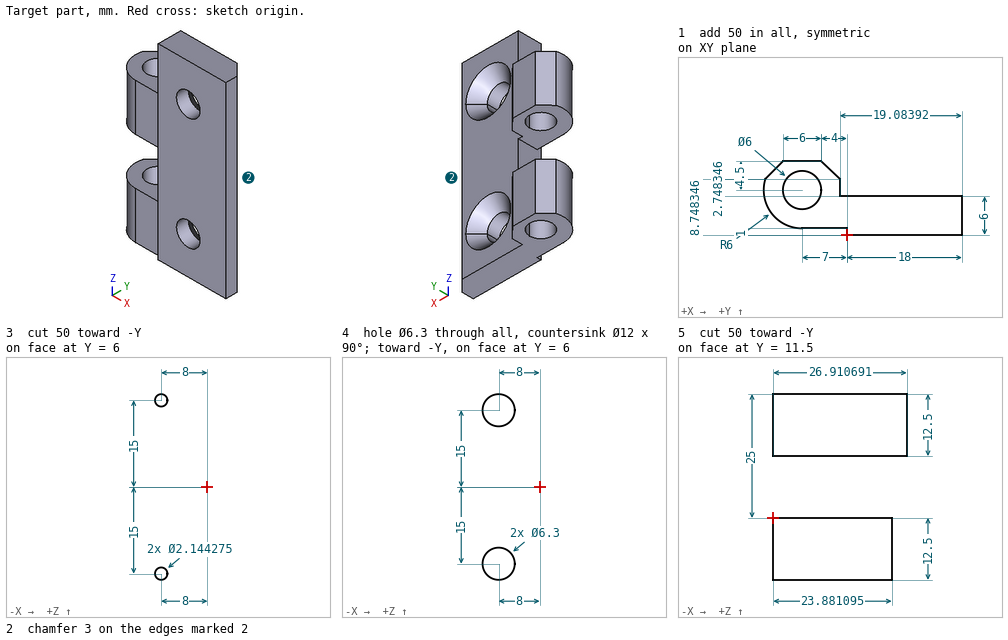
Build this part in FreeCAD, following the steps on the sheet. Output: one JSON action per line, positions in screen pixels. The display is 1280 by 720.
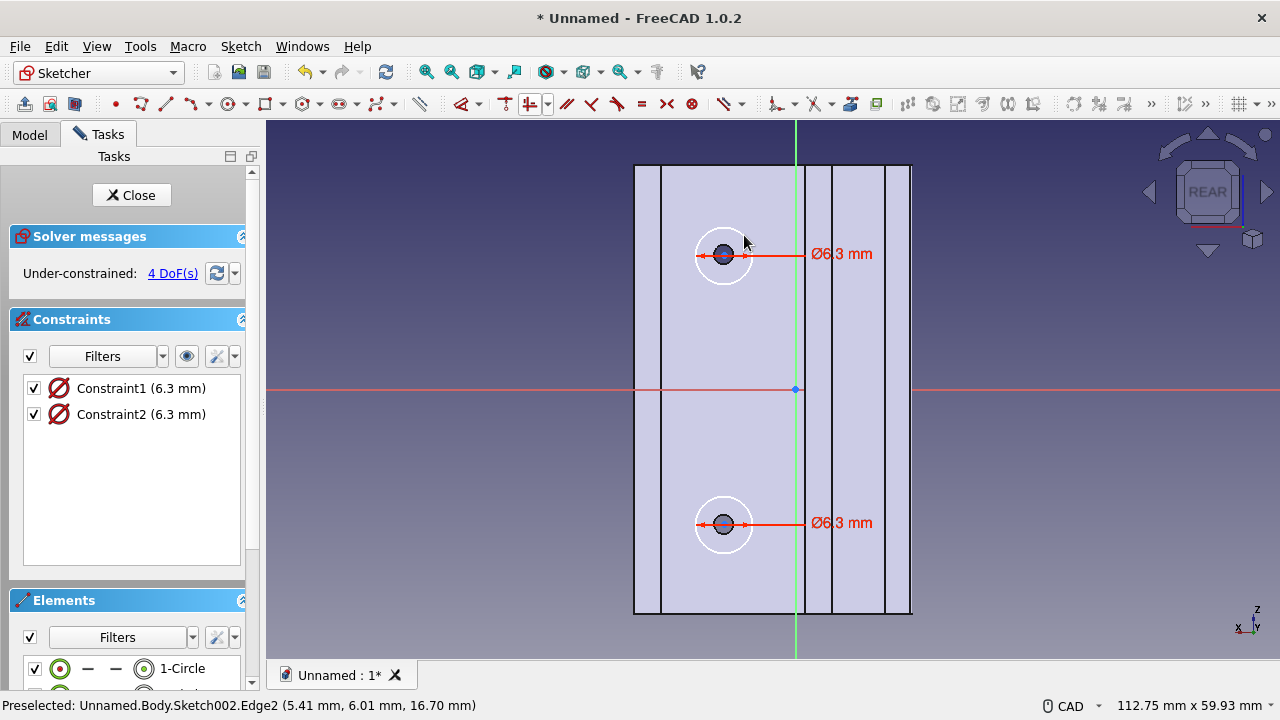
{"action": "left_click", "coordinate": [460, 104]}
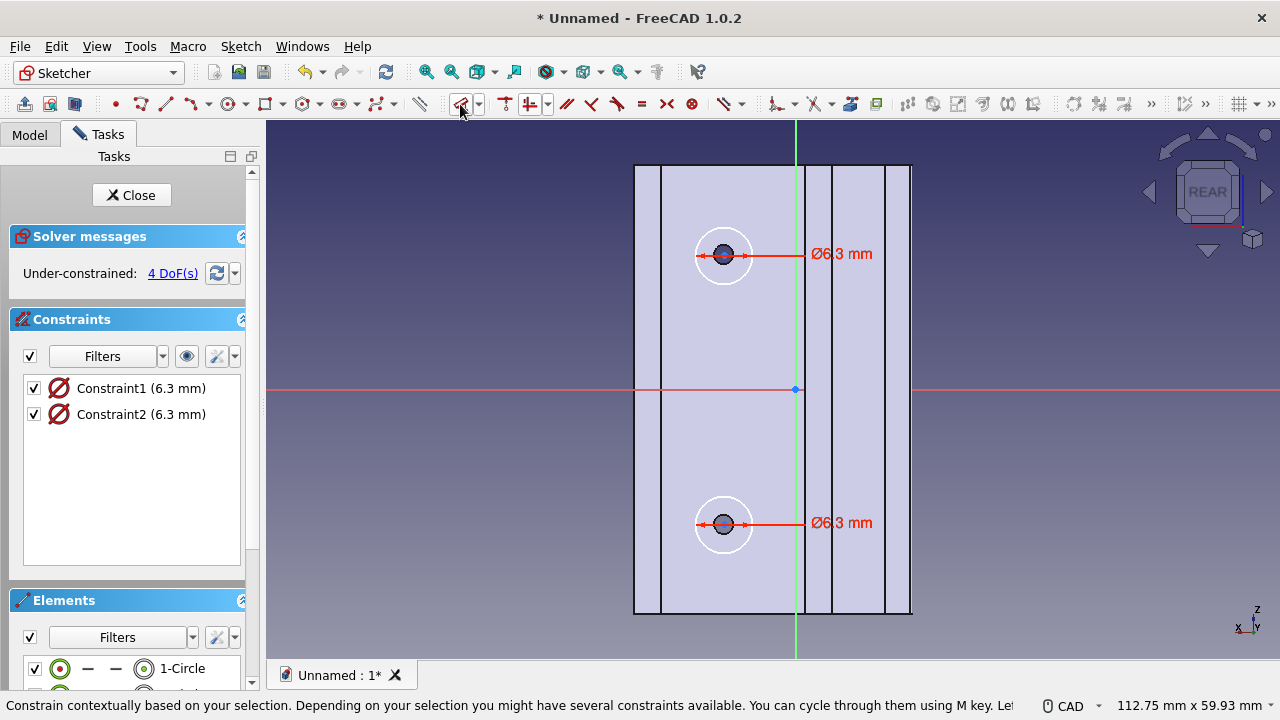
{"action": "left_click", "coordinate": [724, 525]}
{"action": "left_click", "coordinate": [760, 559]}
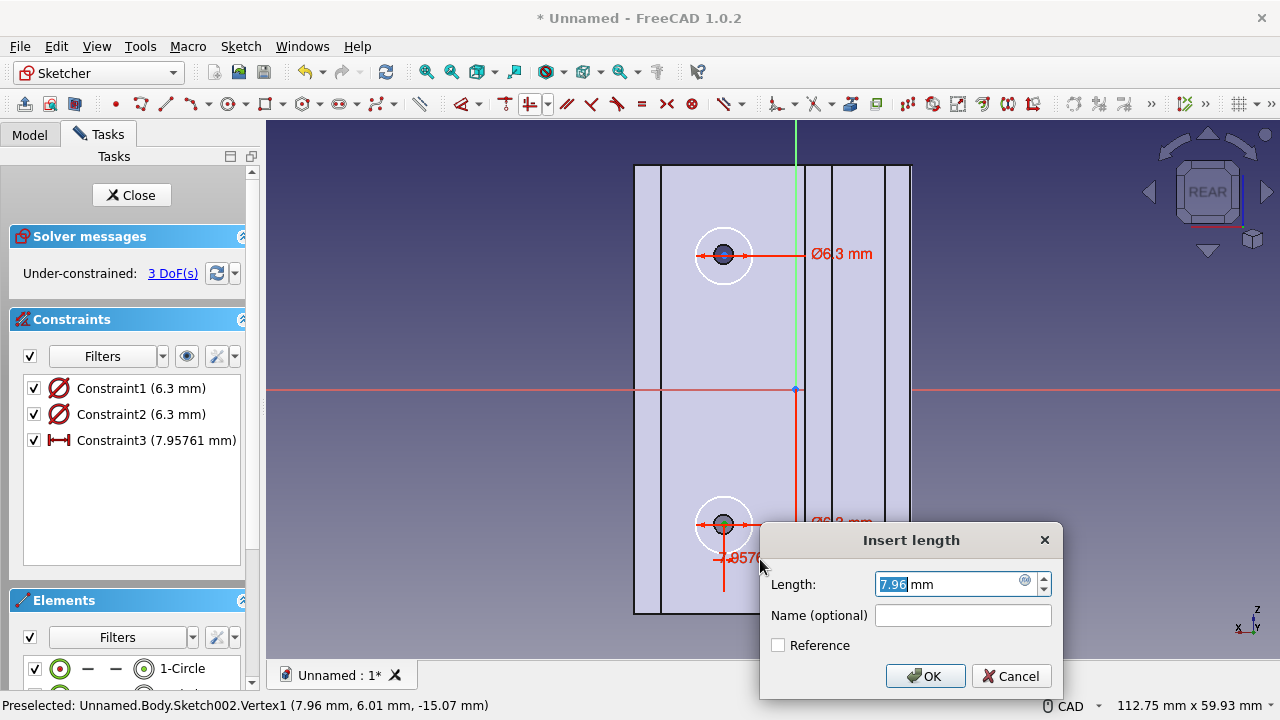
{"action": "type", "text": "8"}
{"action": "key", "text": "Return"}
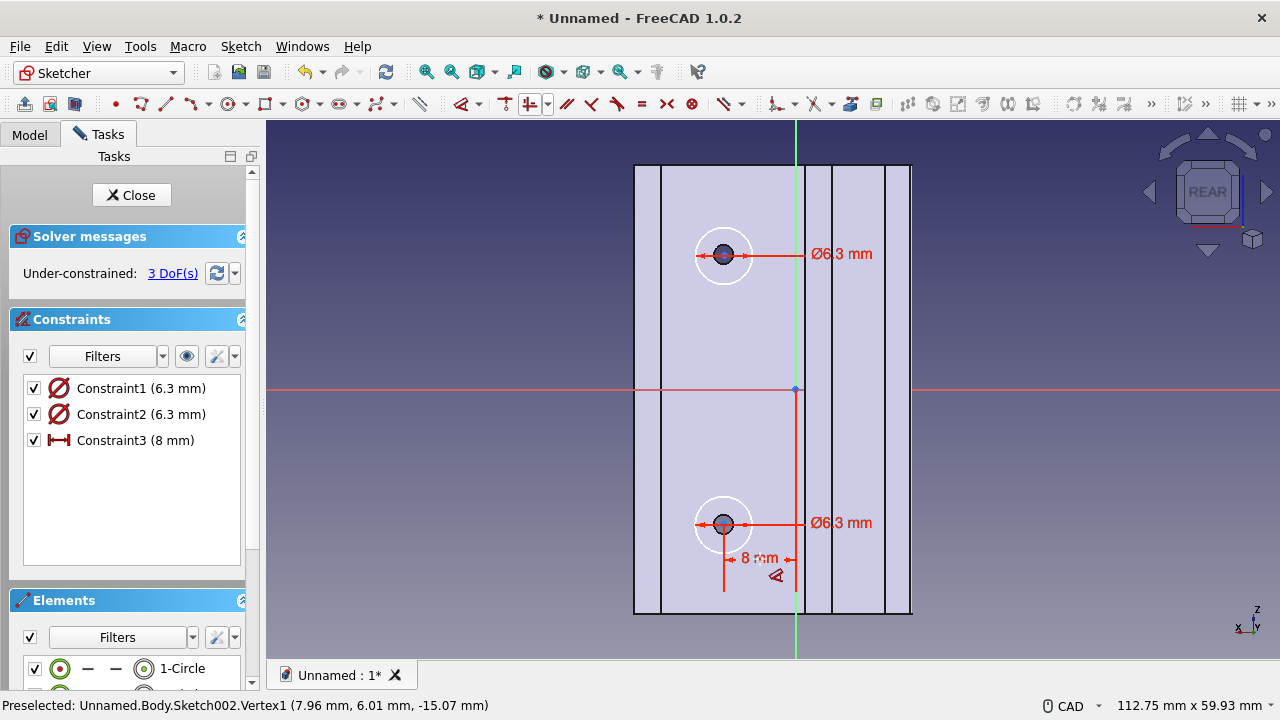
{"action": "left_click", "coordinate": [724, 256]}
{"action": "left_click", "coordinate": [760, 222]}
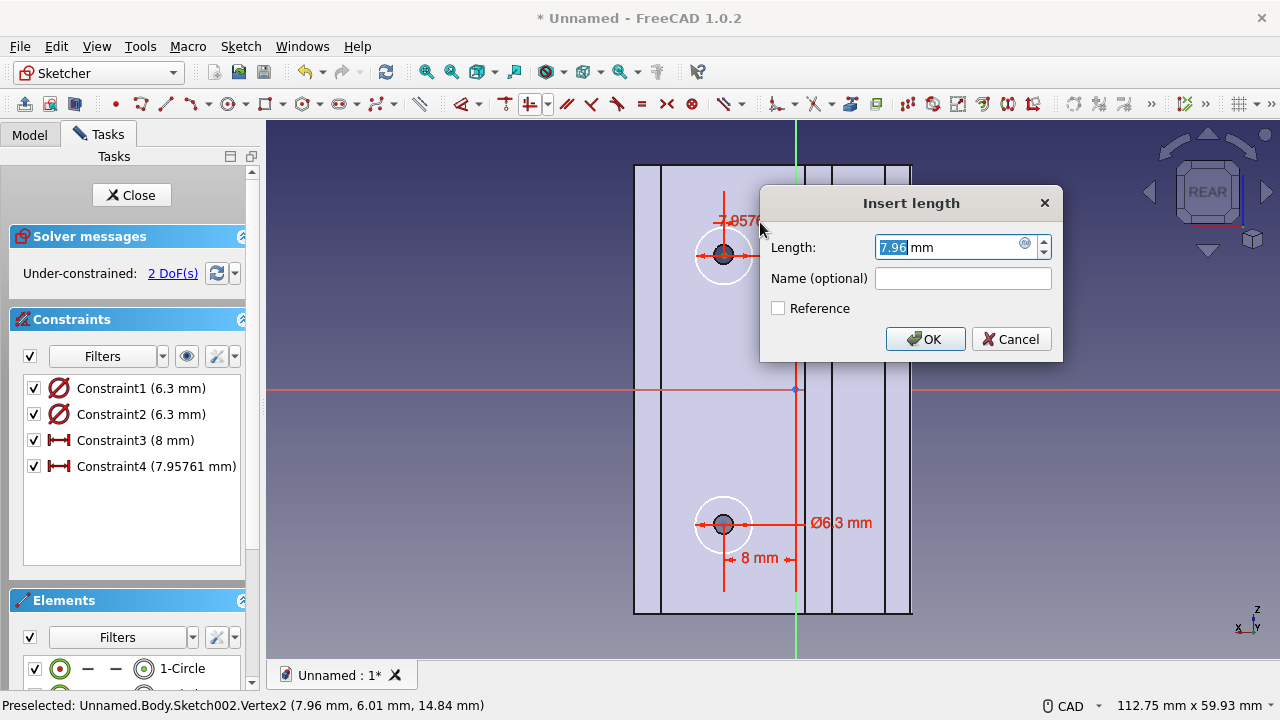
{"action": "type", "text": "8"}
{"action": "key", "text": "Return"}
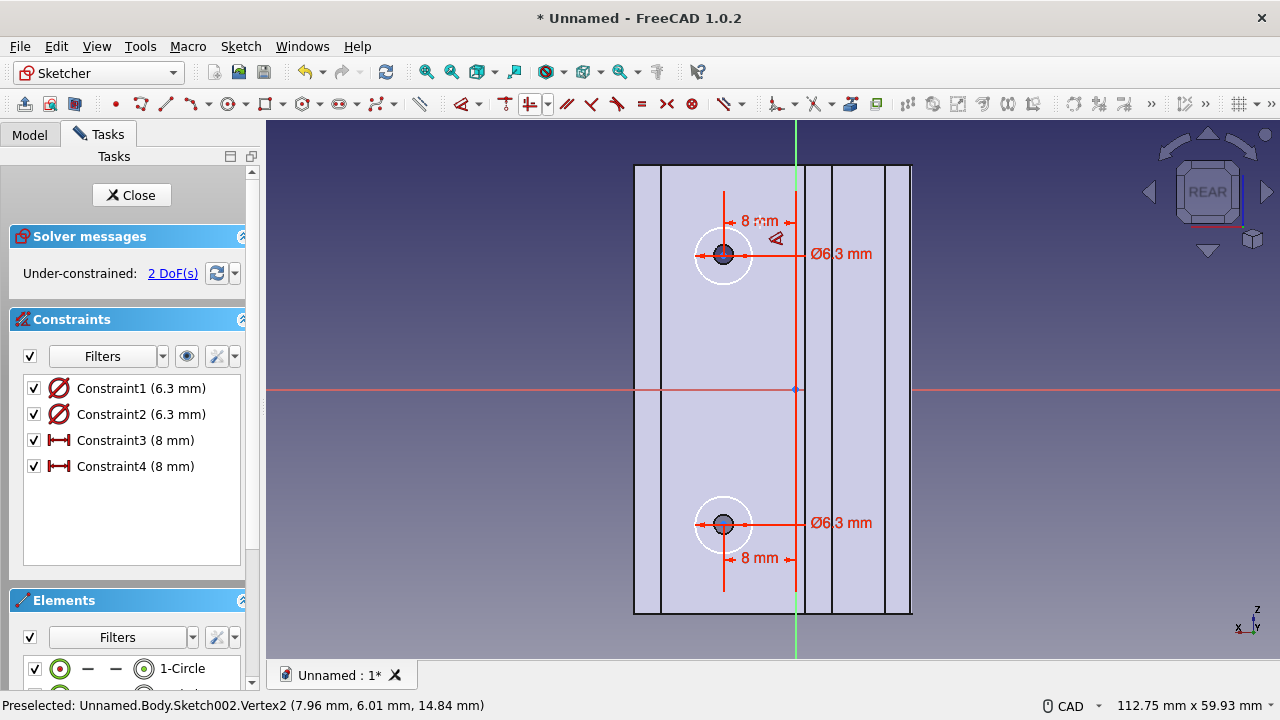
{"action": "left_click", "coordinate": [724, 525]}
{"action": "left_click", "coordinate": [830, 457]}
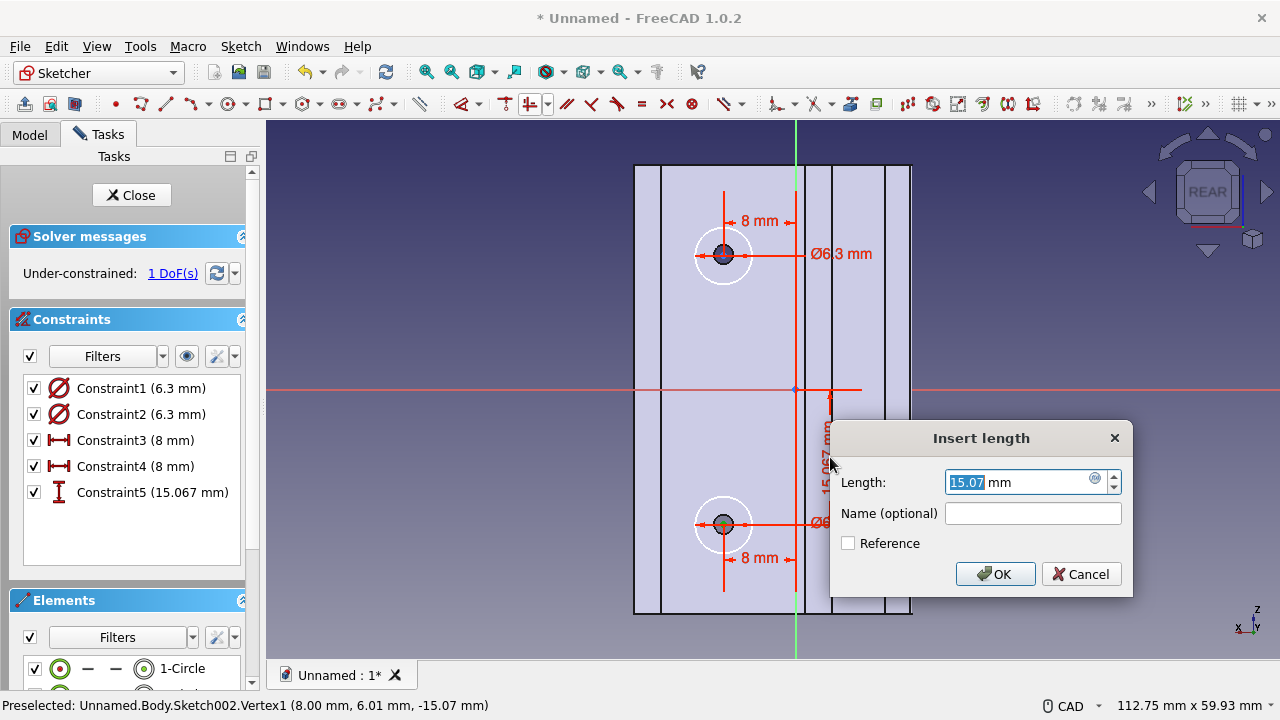
{"action": "type", "text": "15"}
{"action": "key", "text": "Return"}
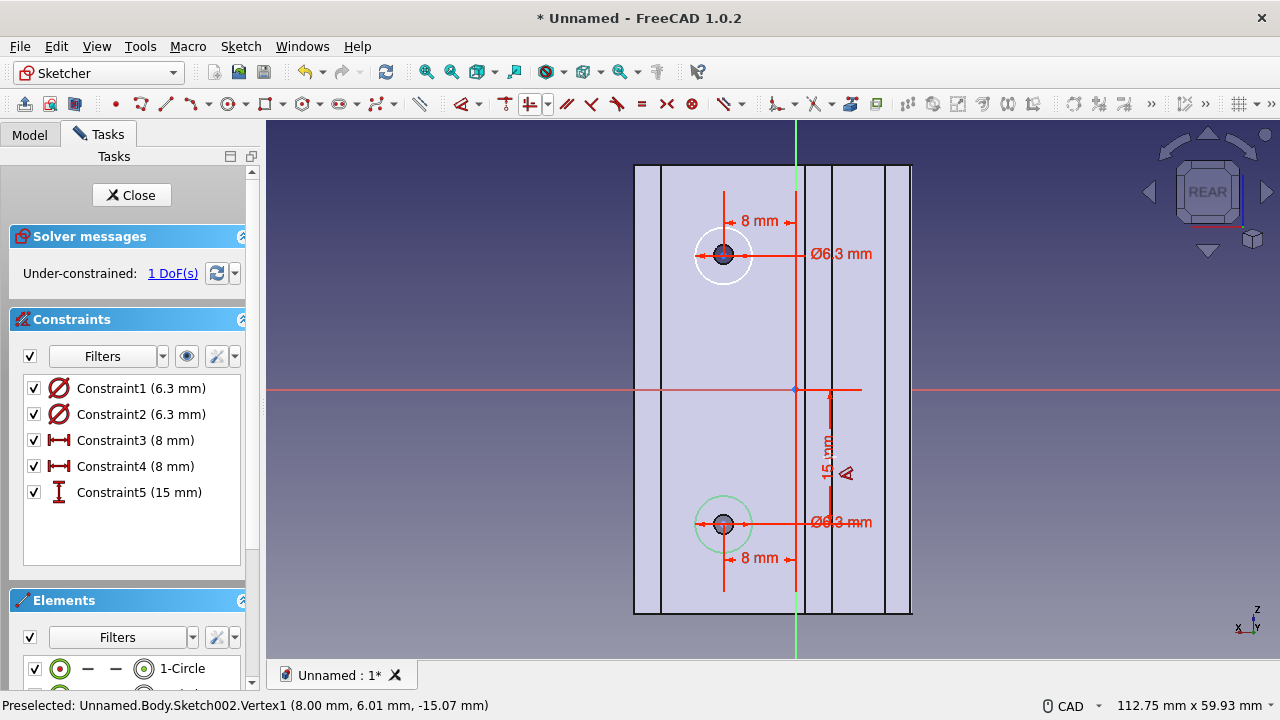
{"action": "left_click", "coordinate": [724, 256]}
{"action": "left_click", "coordinate": [830, 323]}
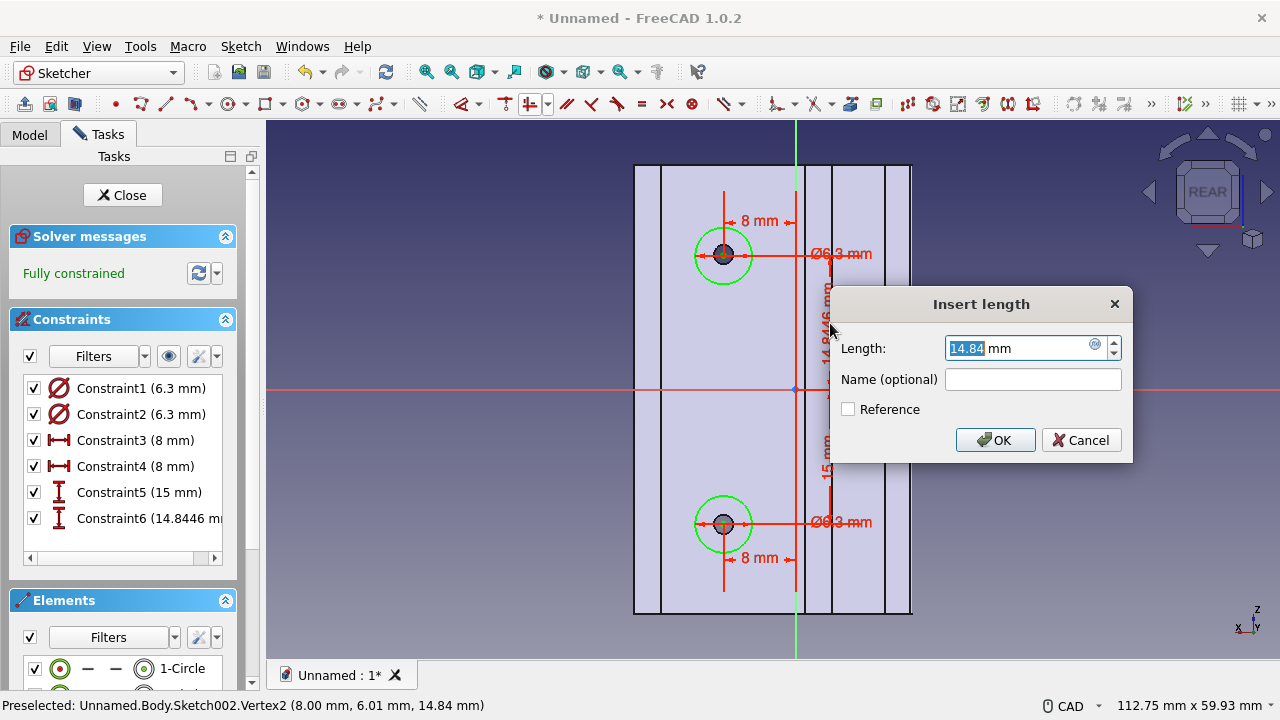
{"action": "type", "text": "15"}
{"action": "key", "text": "Return"}
{"action": "key", "text": "Escape"}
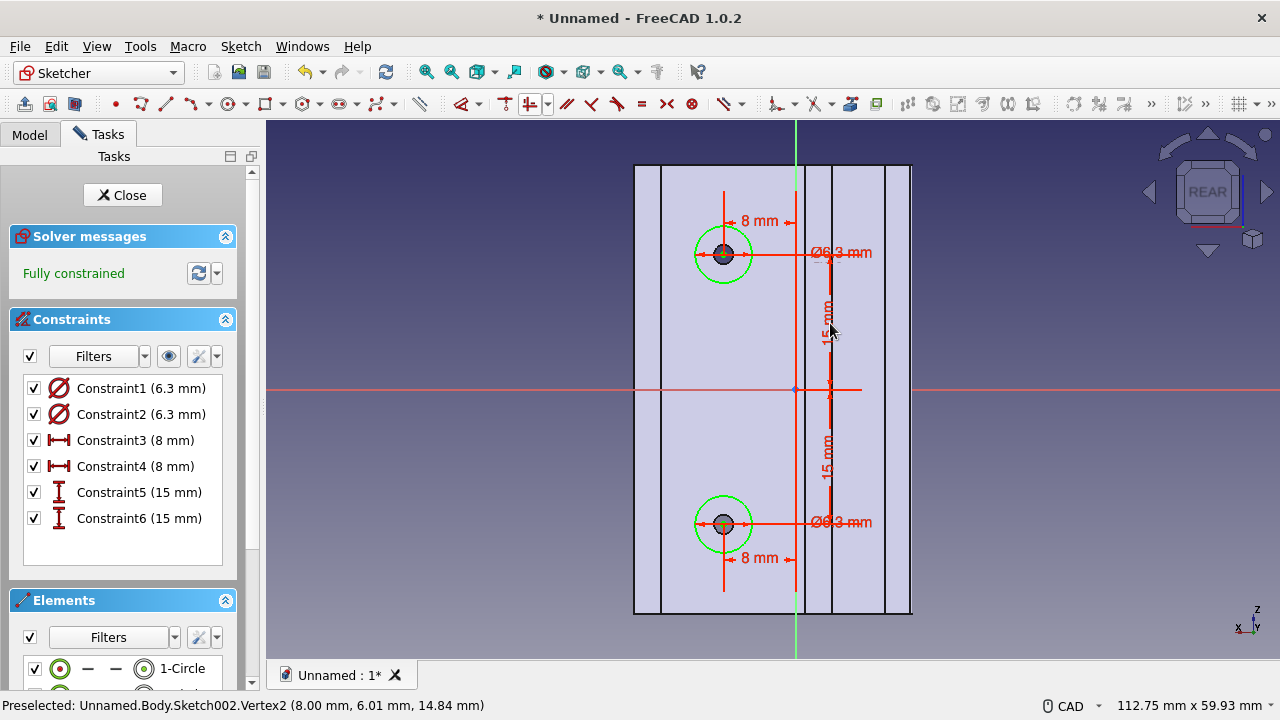
{"action": "left_click", "coordinate": [123, 195]}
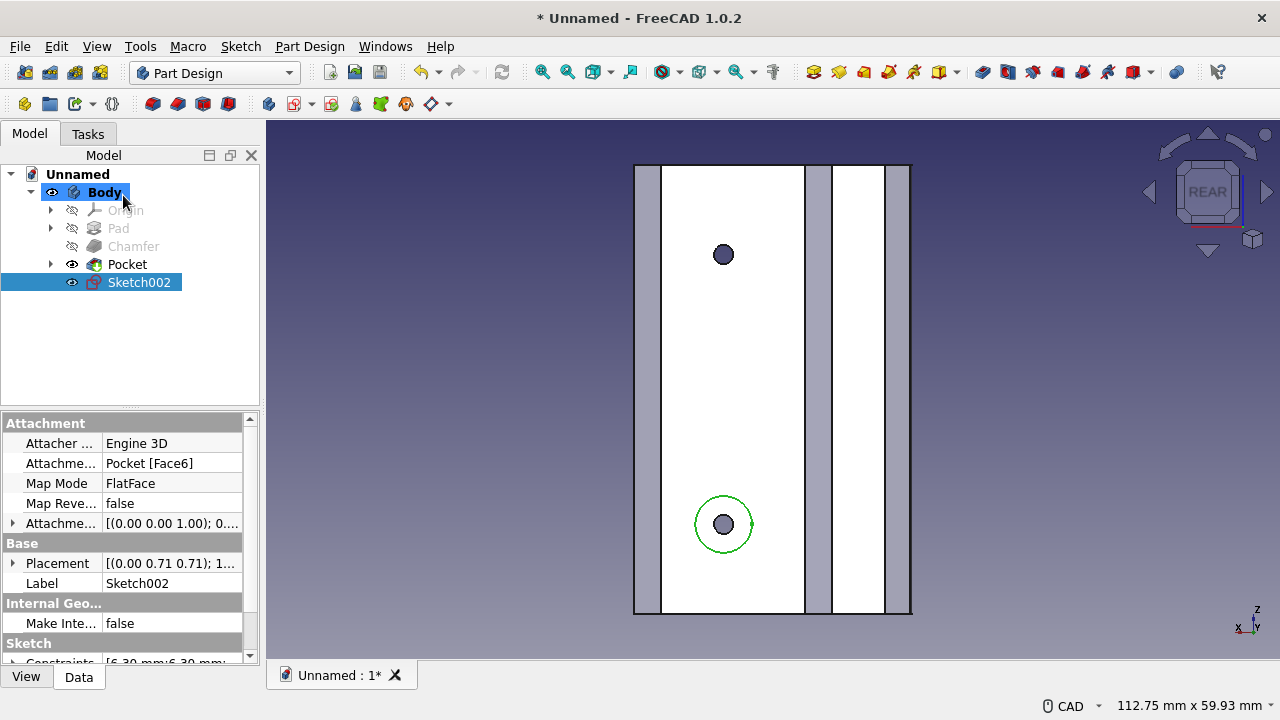
{"action": "left_click", "coordinate": [1008, 72]}